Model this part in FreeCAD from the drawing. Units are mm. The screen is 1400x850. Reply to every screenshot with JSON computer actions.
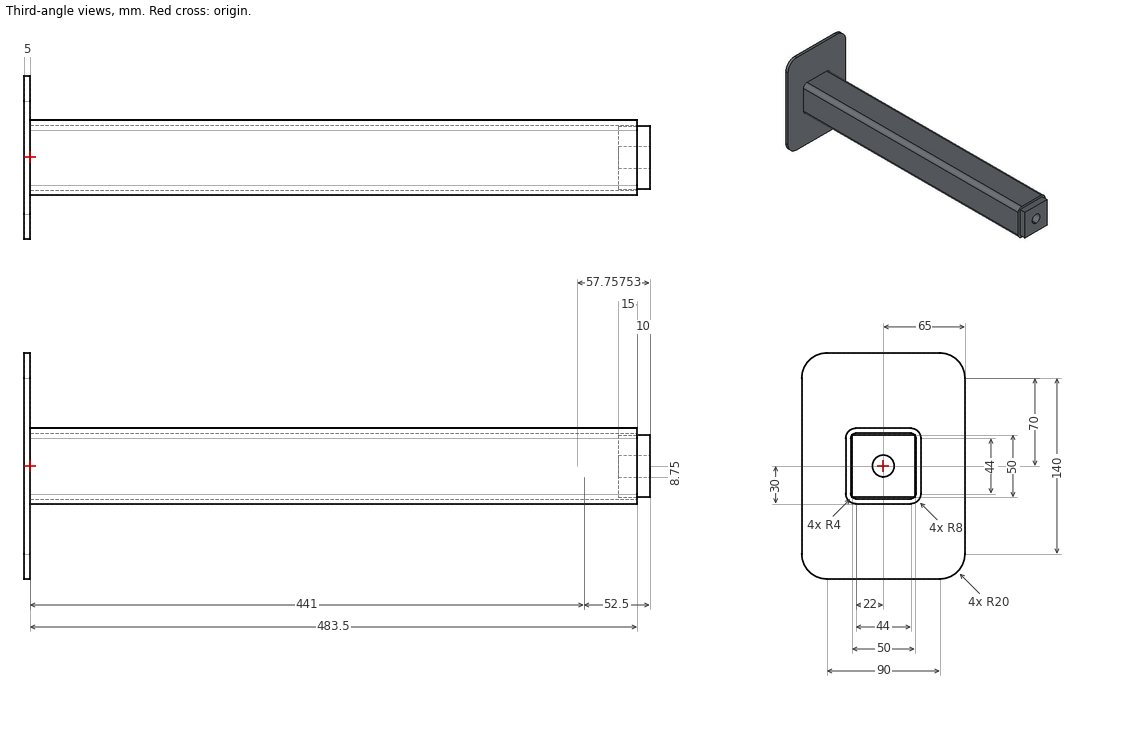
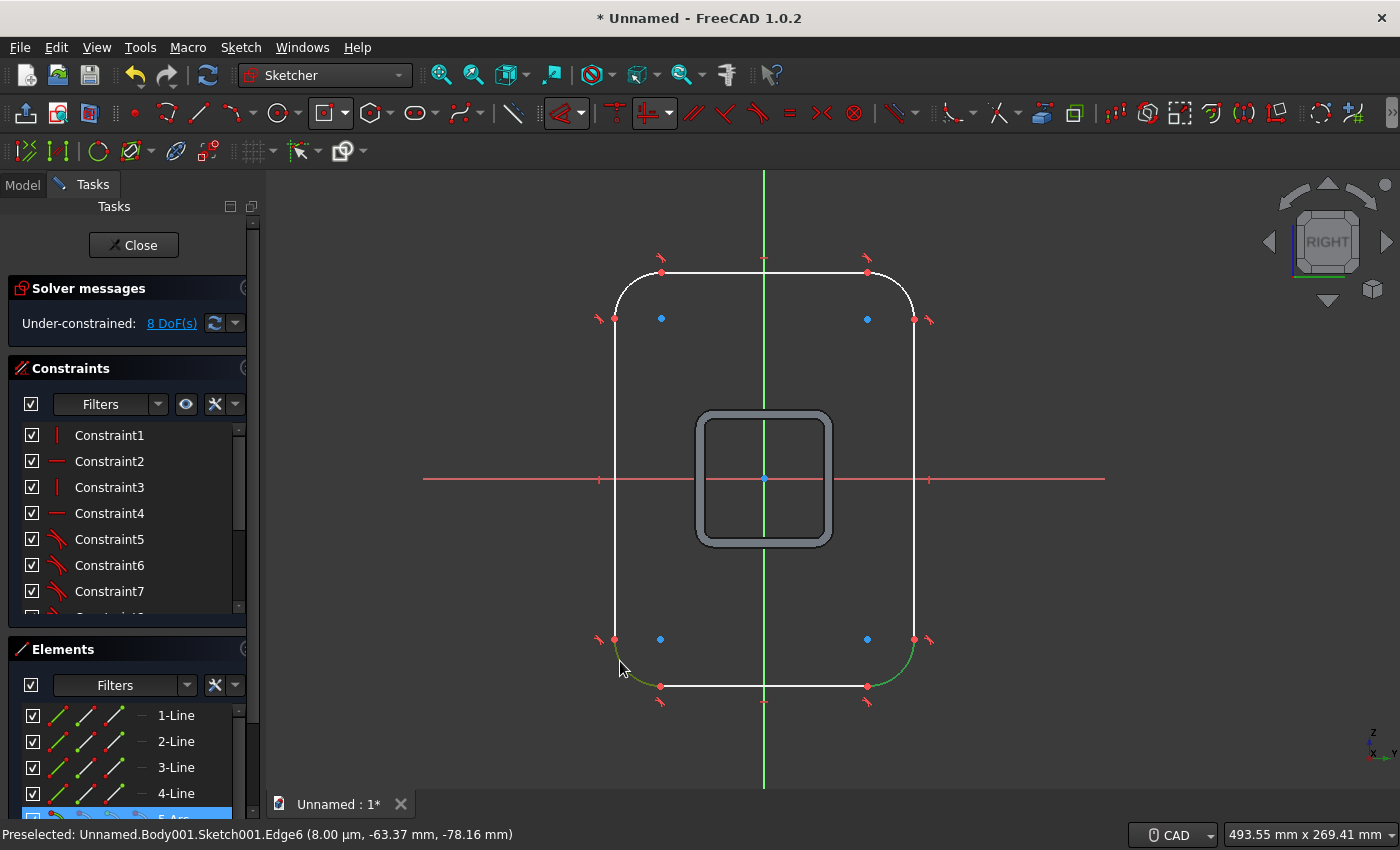
{"action": "left_click", "coordinate": [640, 278]}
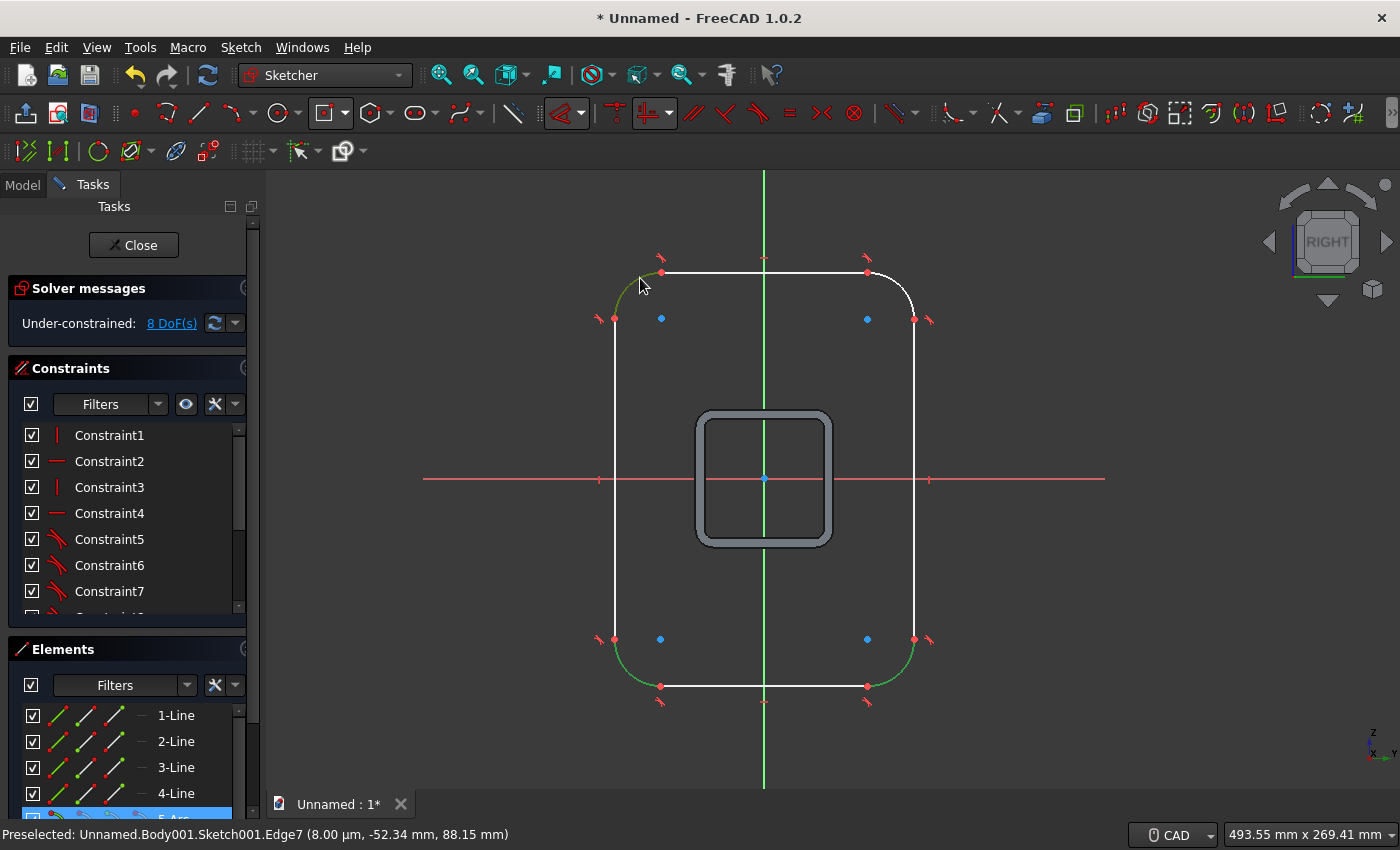
{"action": "left_click", "coordinate": [909, 298]}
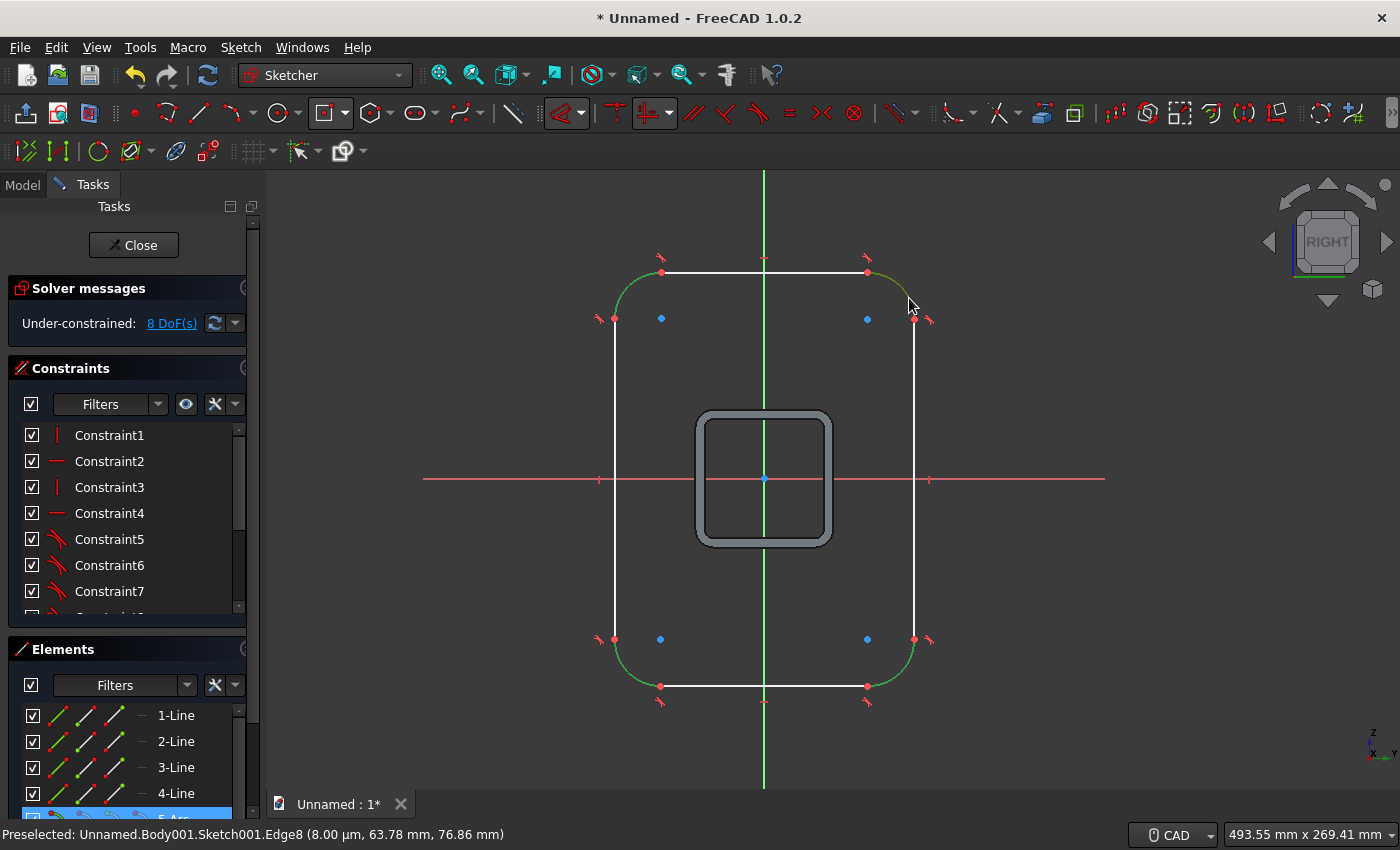
{"action": "left_click", "coordinate": [790, 114]}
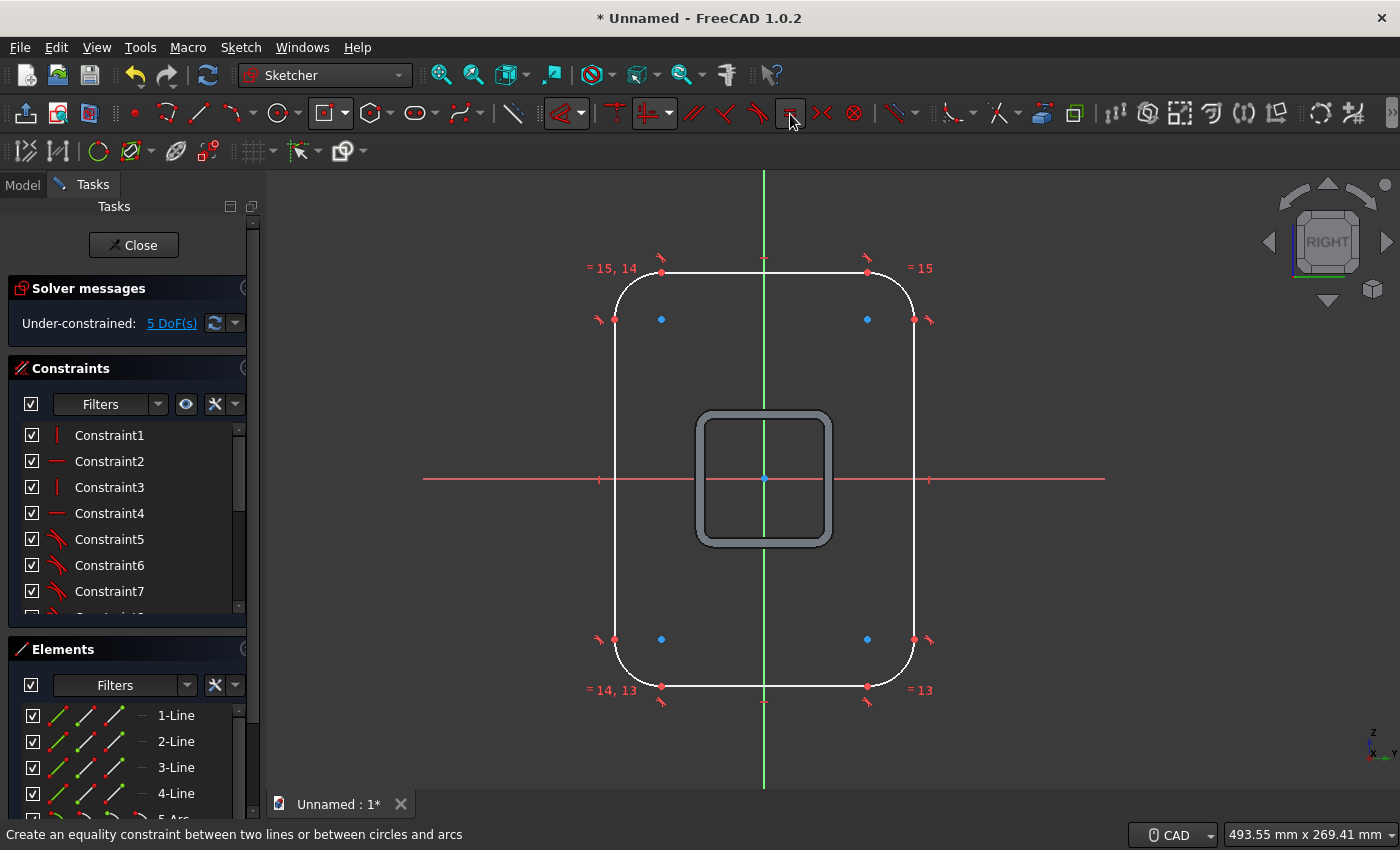
{"action": "left_click", "coordinate": [889, 681]}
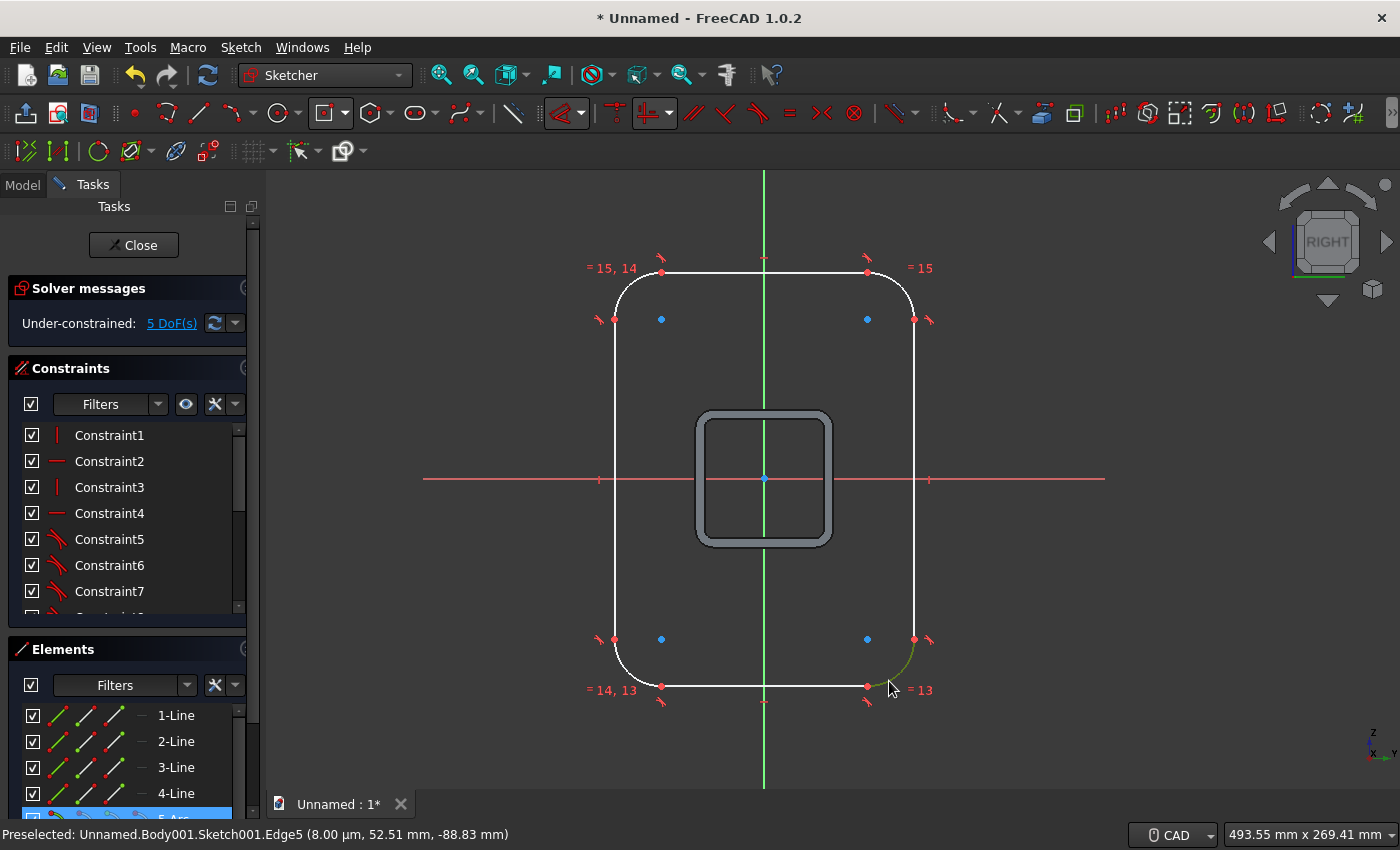
{"action": "key", "text": "k r"}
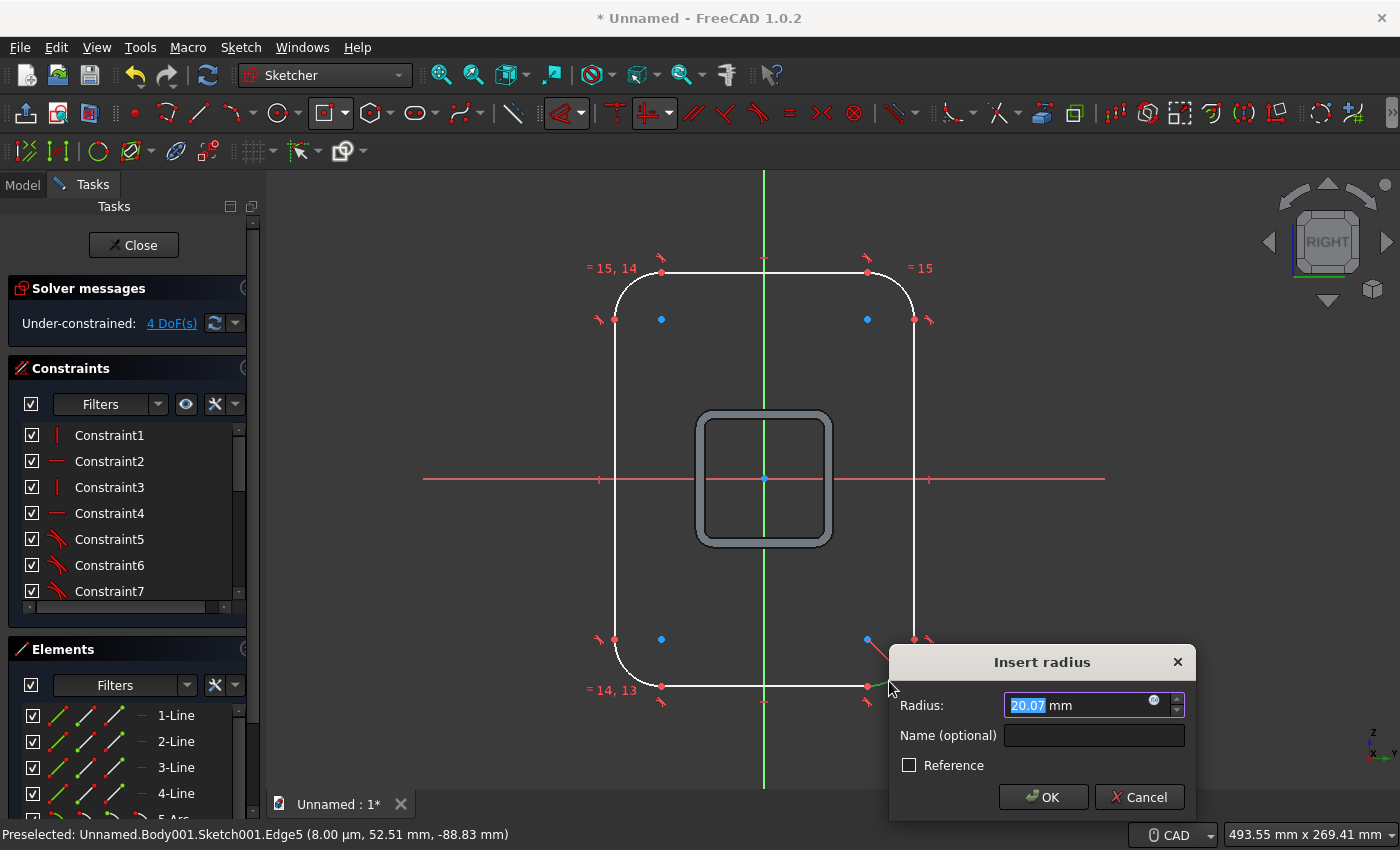
{"action": "type", "text": "20"}
{"action": "key", "text": "Return"}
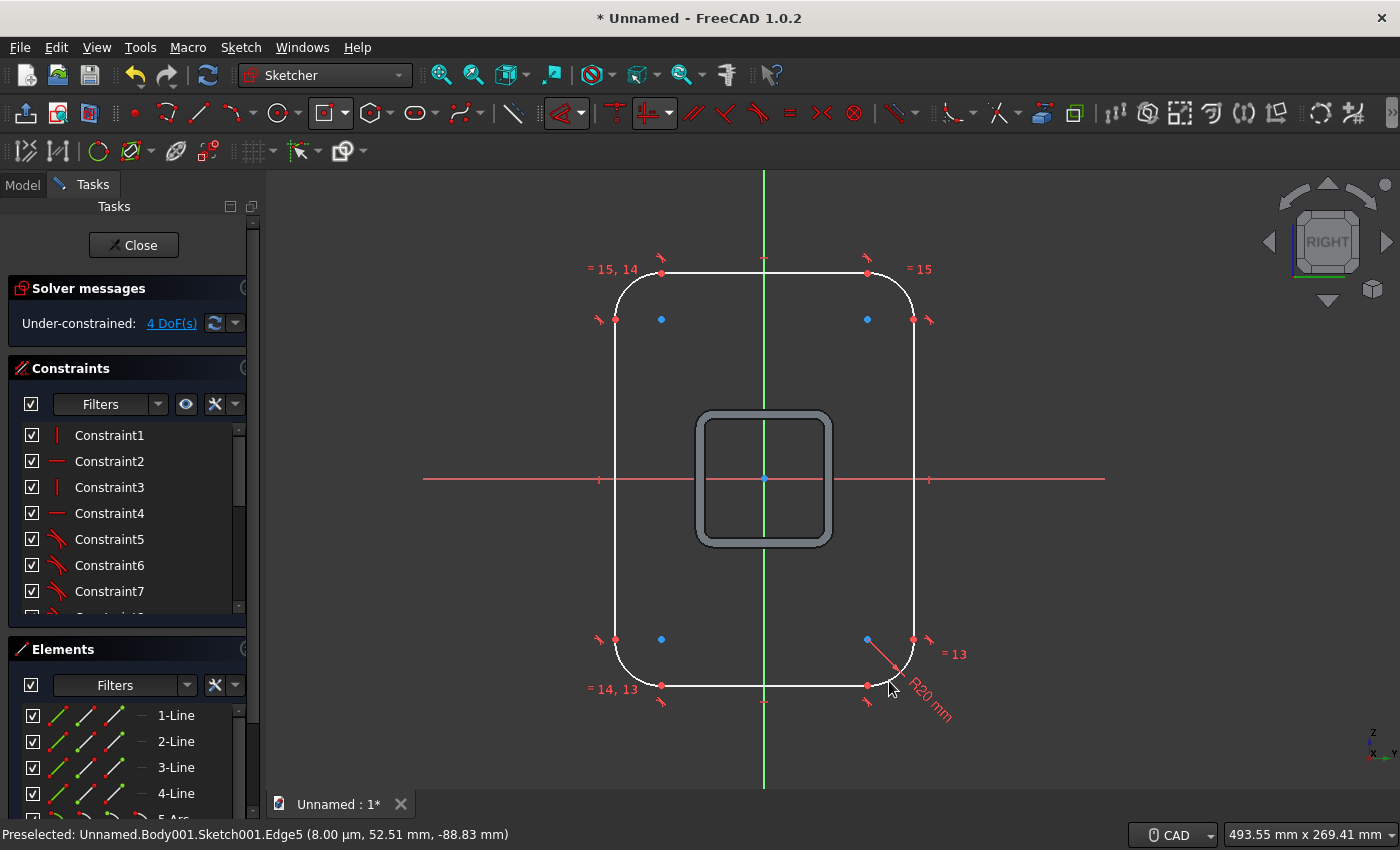
{"action": "left_click", "coordinate": [806, 686]}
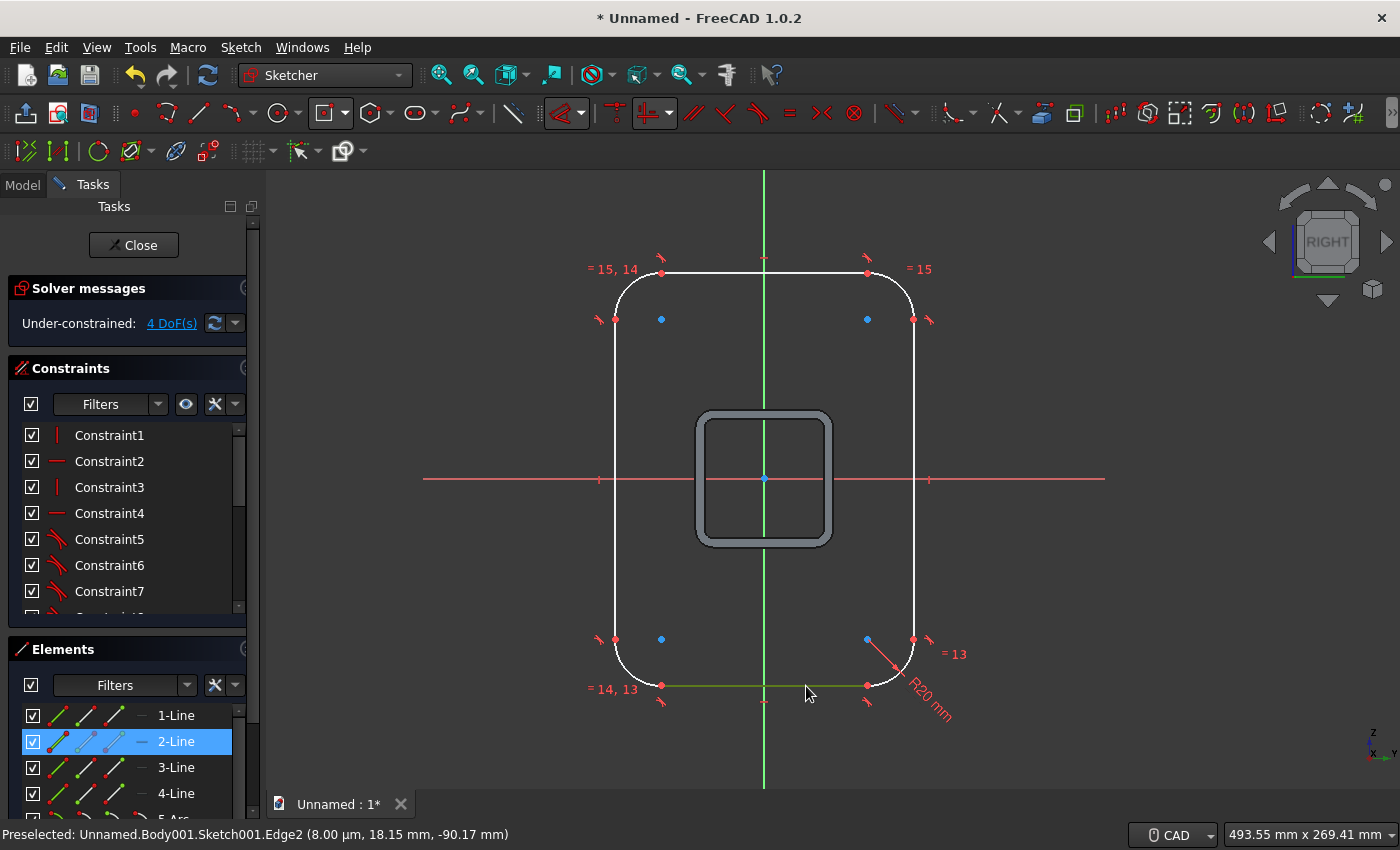
{"action": "key", "text": "l"}